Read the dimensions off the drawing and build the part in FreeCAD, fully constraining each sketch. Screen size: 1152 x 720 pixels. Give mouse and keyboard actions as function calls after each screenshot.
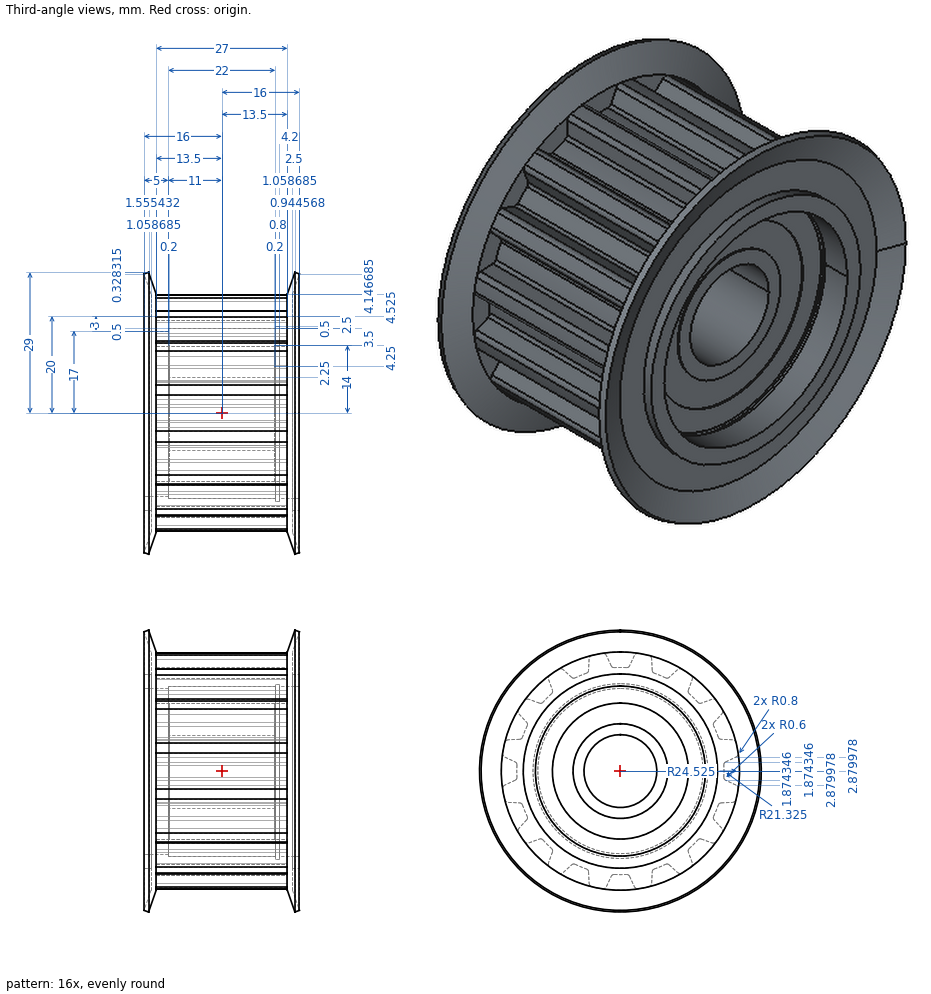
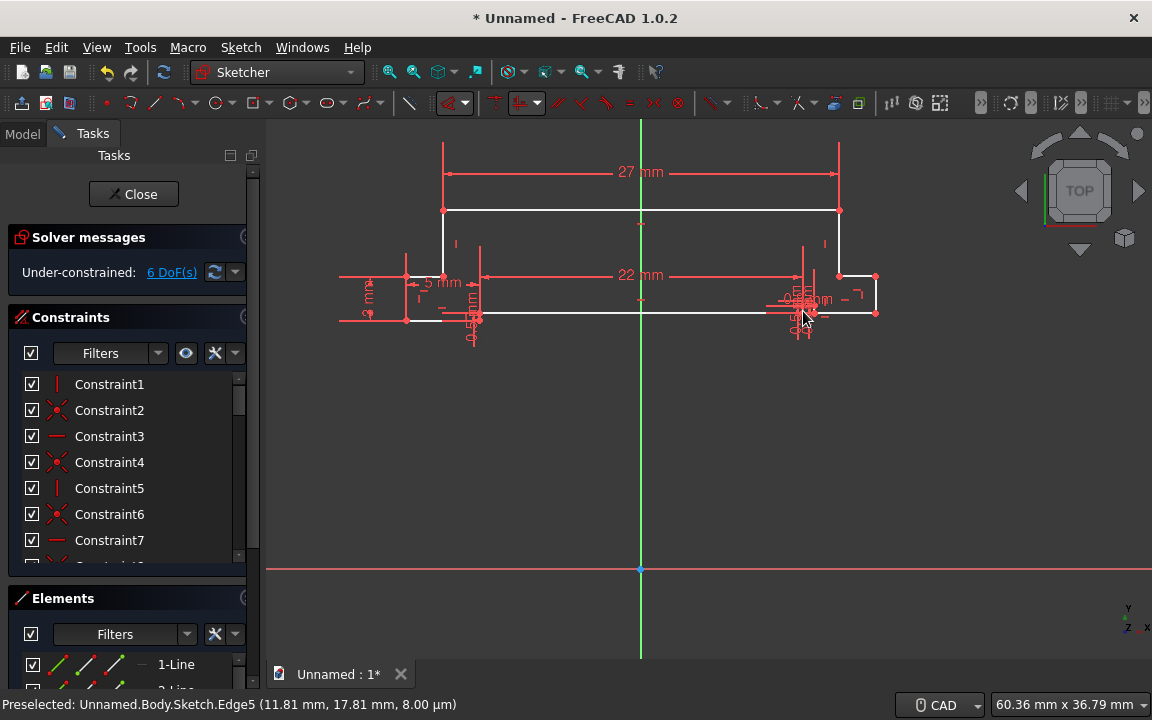
click(857, 313)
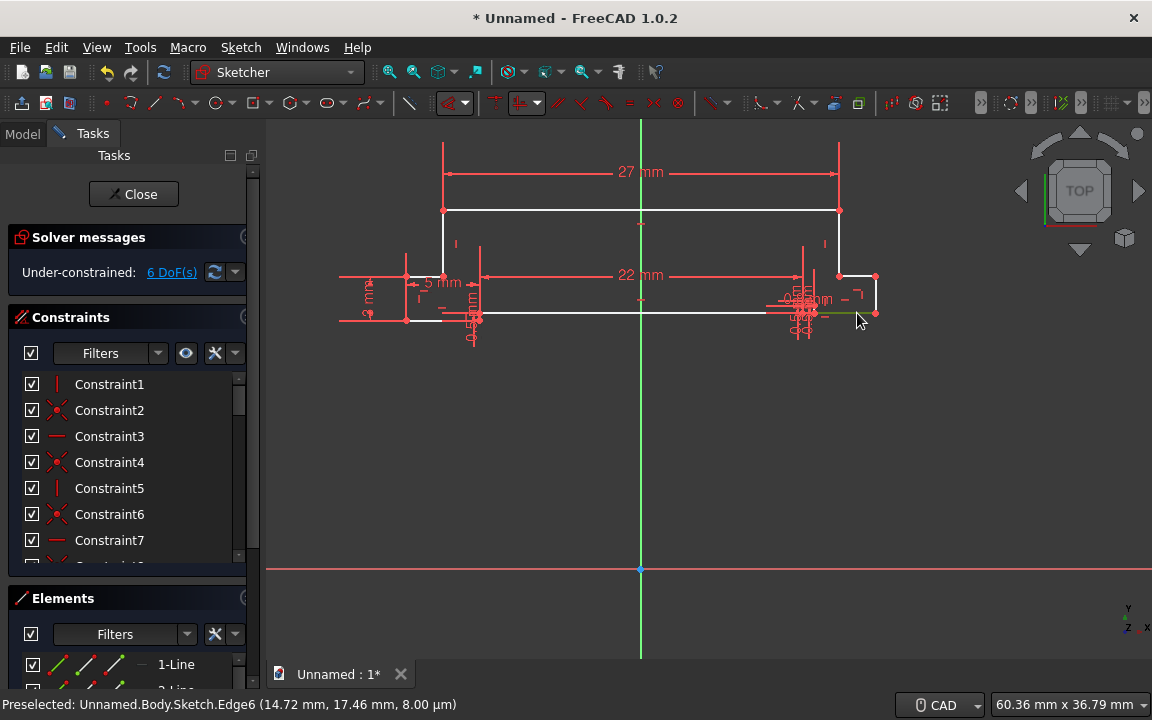
key(l)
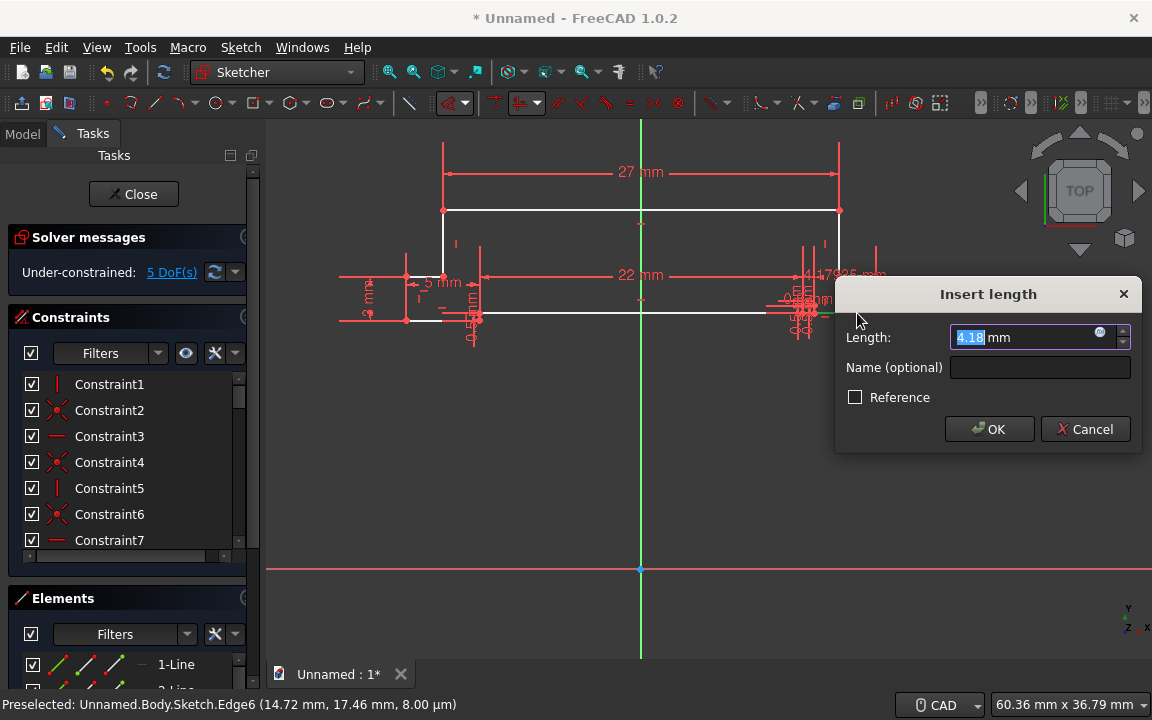
text(4.2)
key(Return)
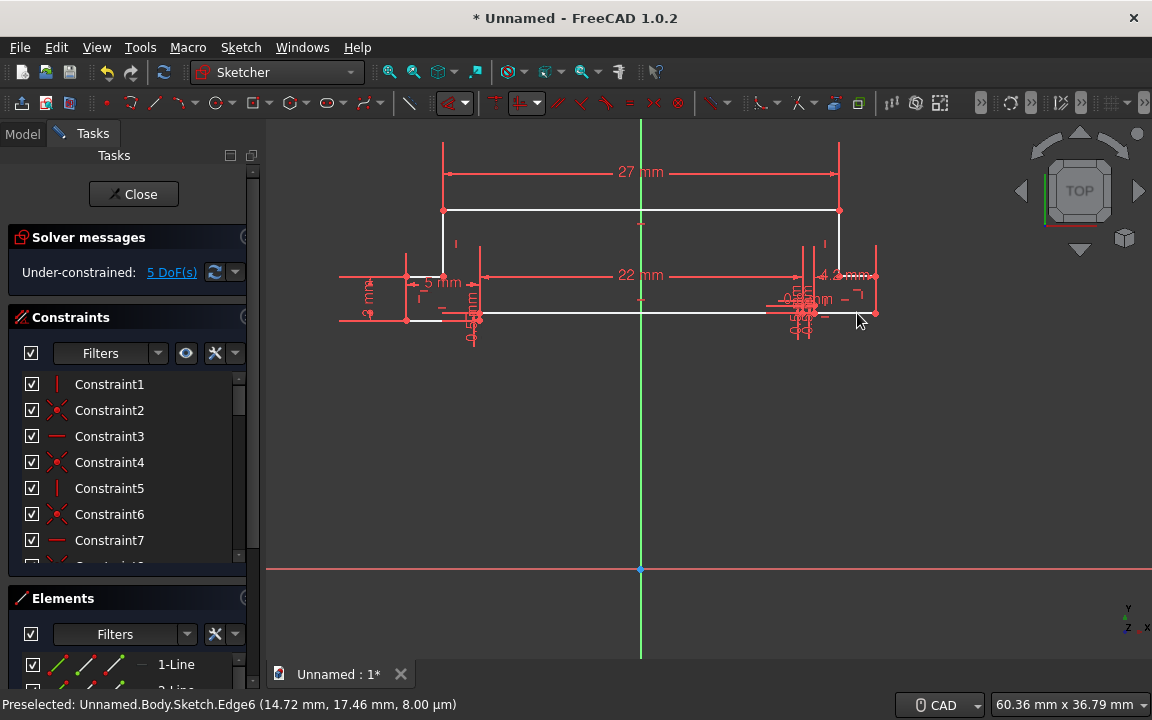
scroll(876, 302, up, 2)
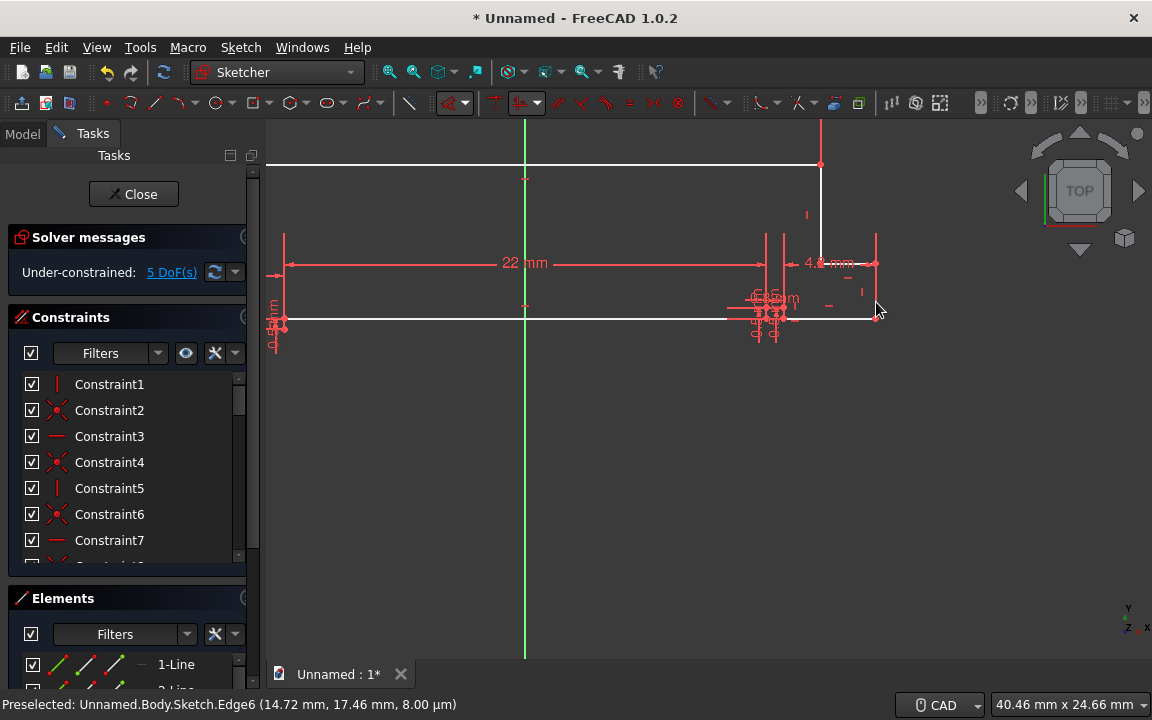
click(876, 302)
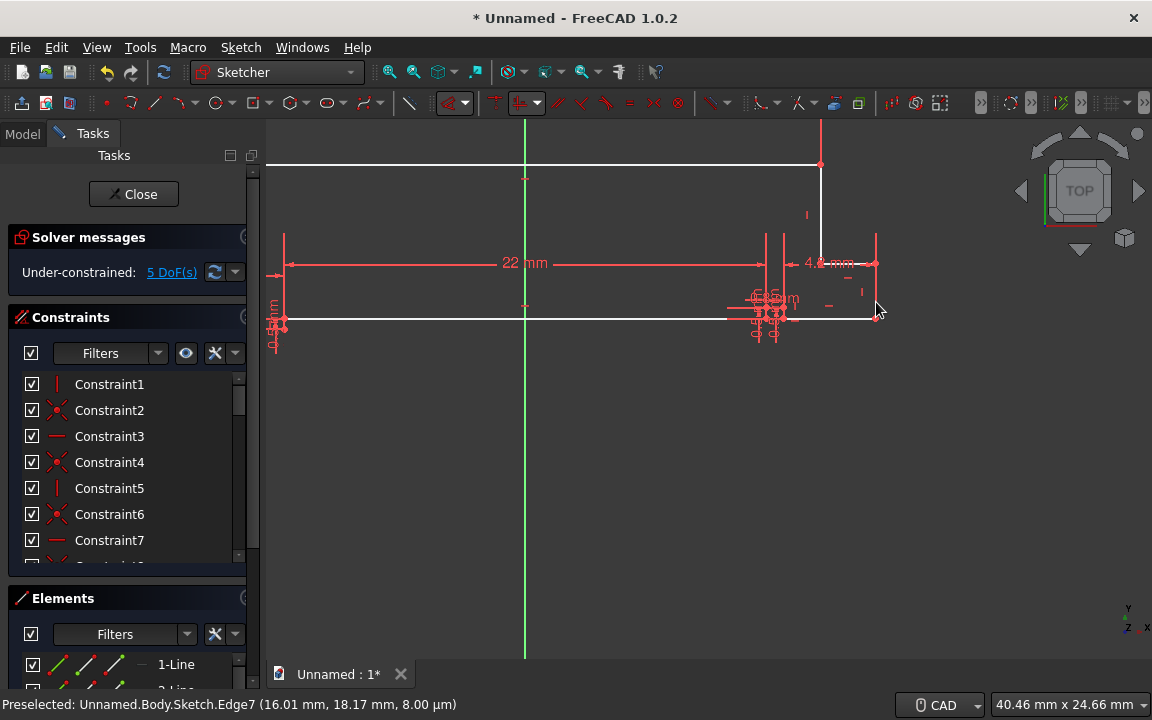
key(i)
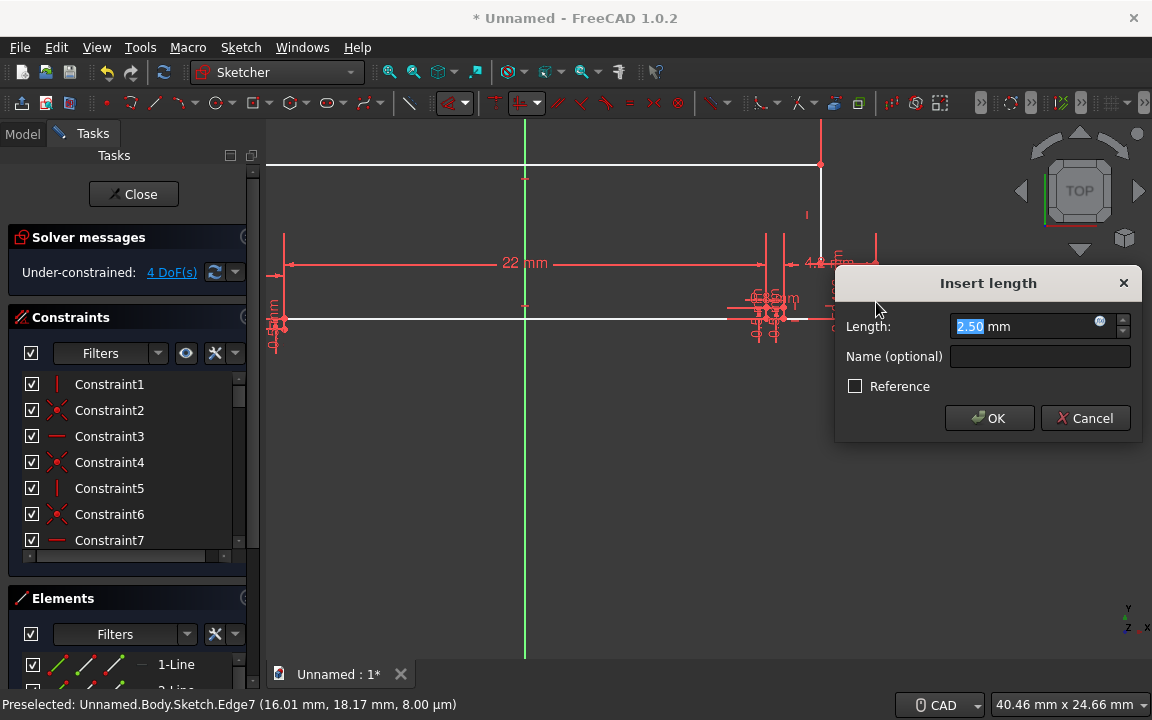
text(2.5)
key(Return)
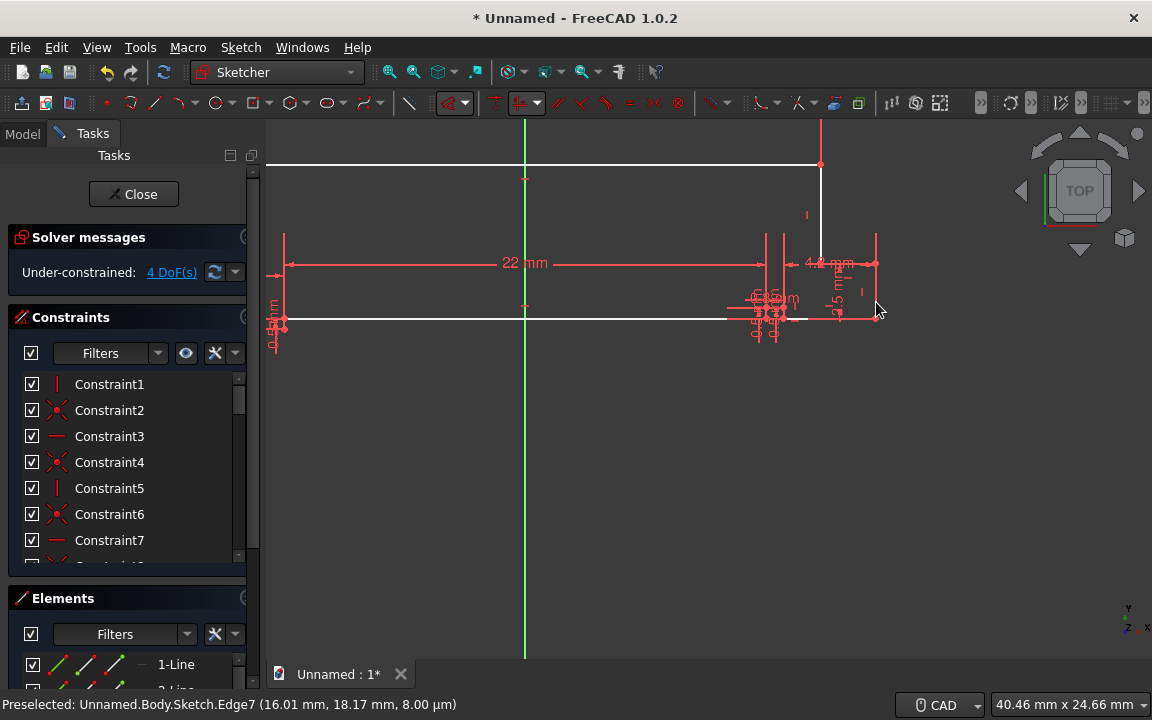
click(859, 264)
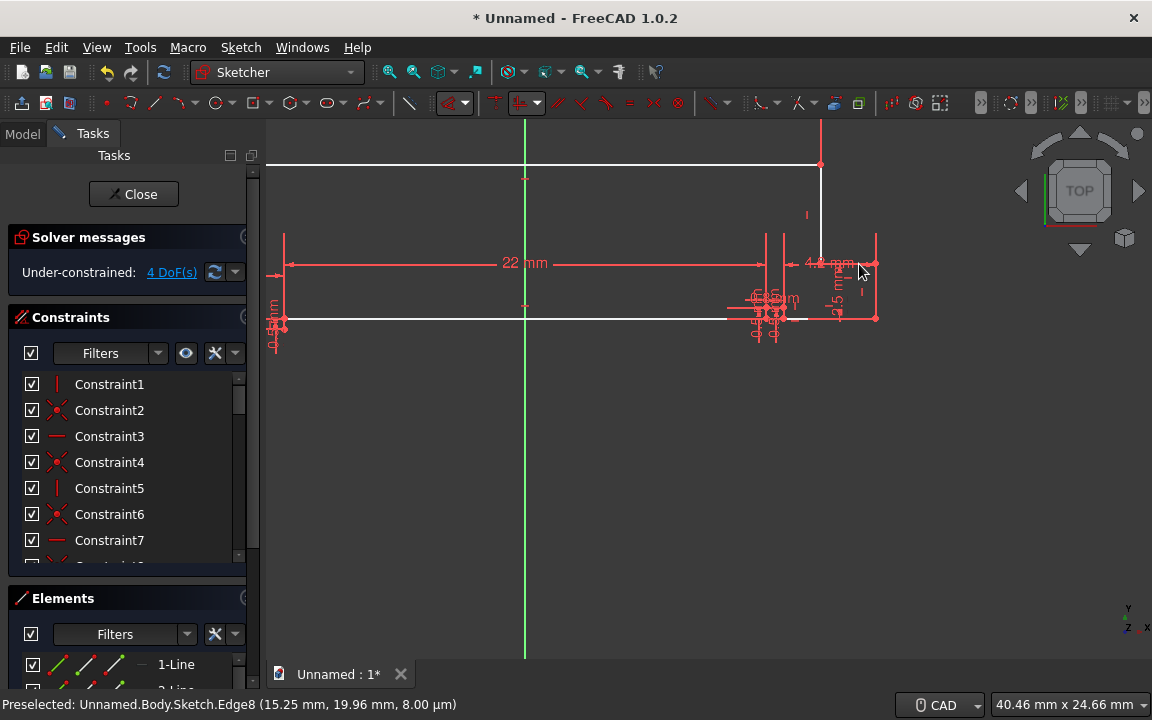
click(468, 104)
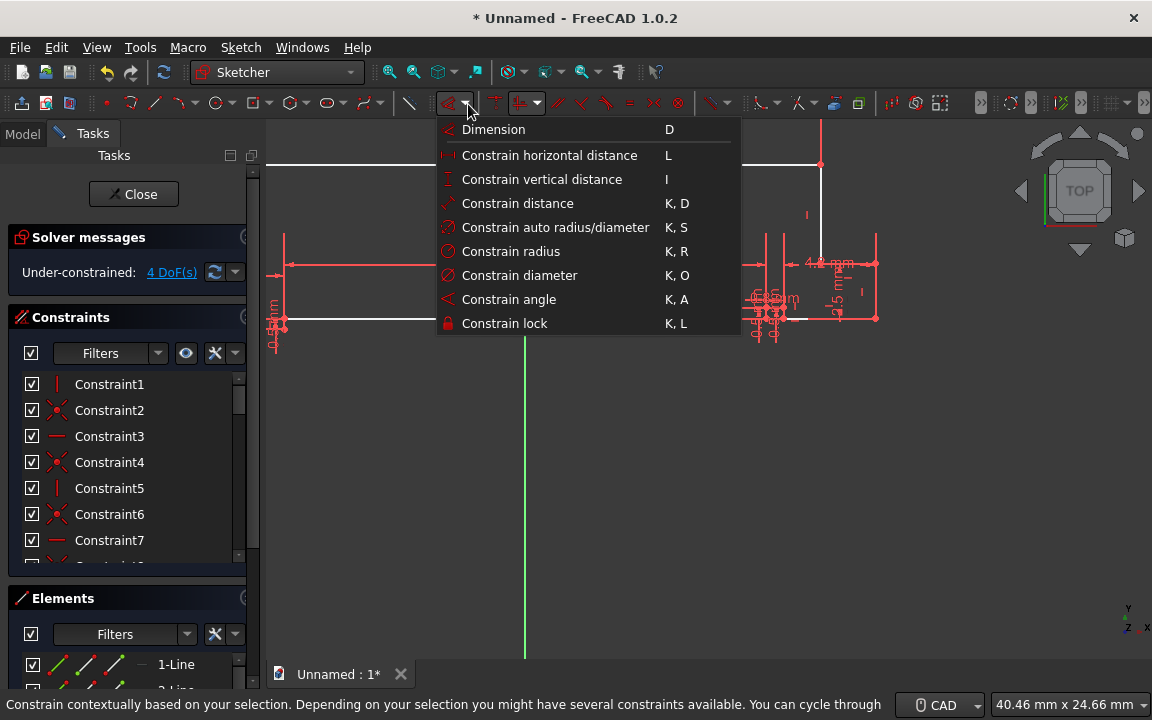
click(589, 155)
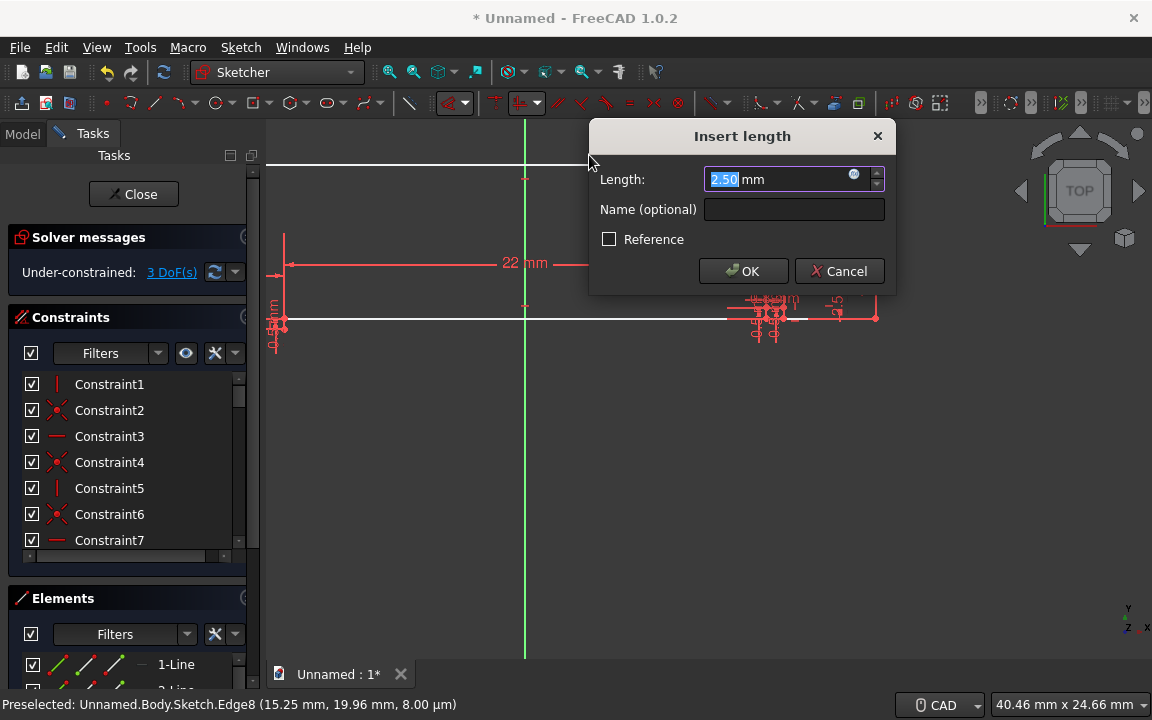
text(2.5)
key(Return)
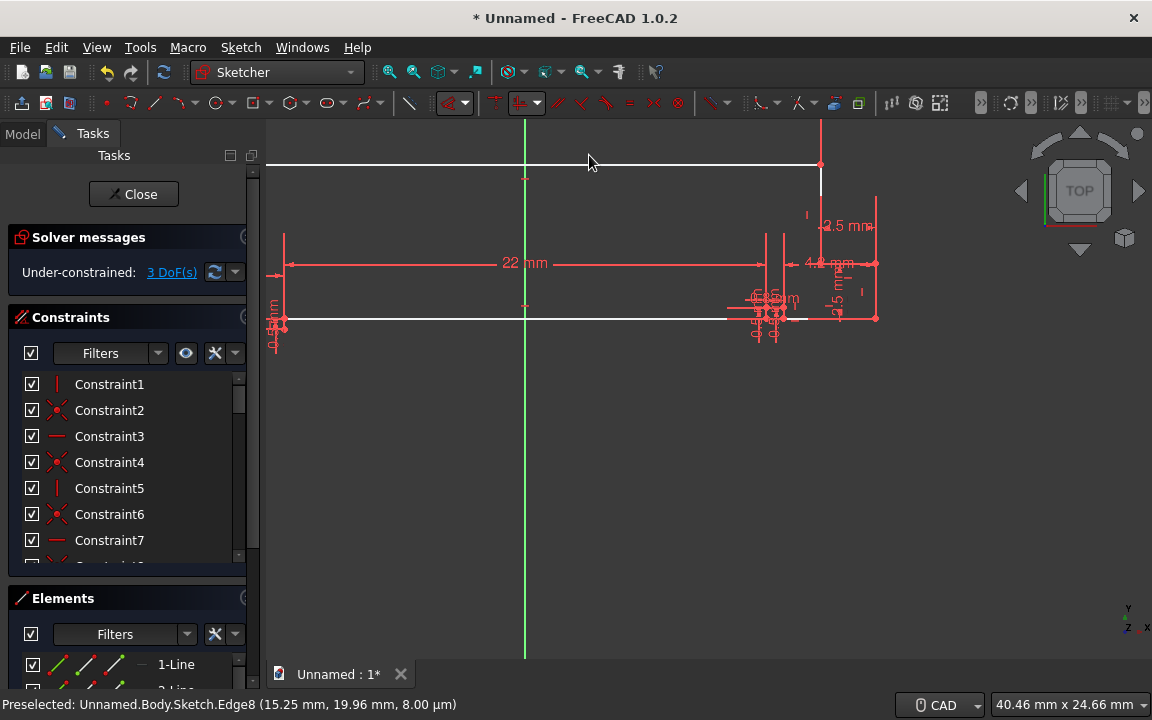
scroll(875, 301, down, 2)